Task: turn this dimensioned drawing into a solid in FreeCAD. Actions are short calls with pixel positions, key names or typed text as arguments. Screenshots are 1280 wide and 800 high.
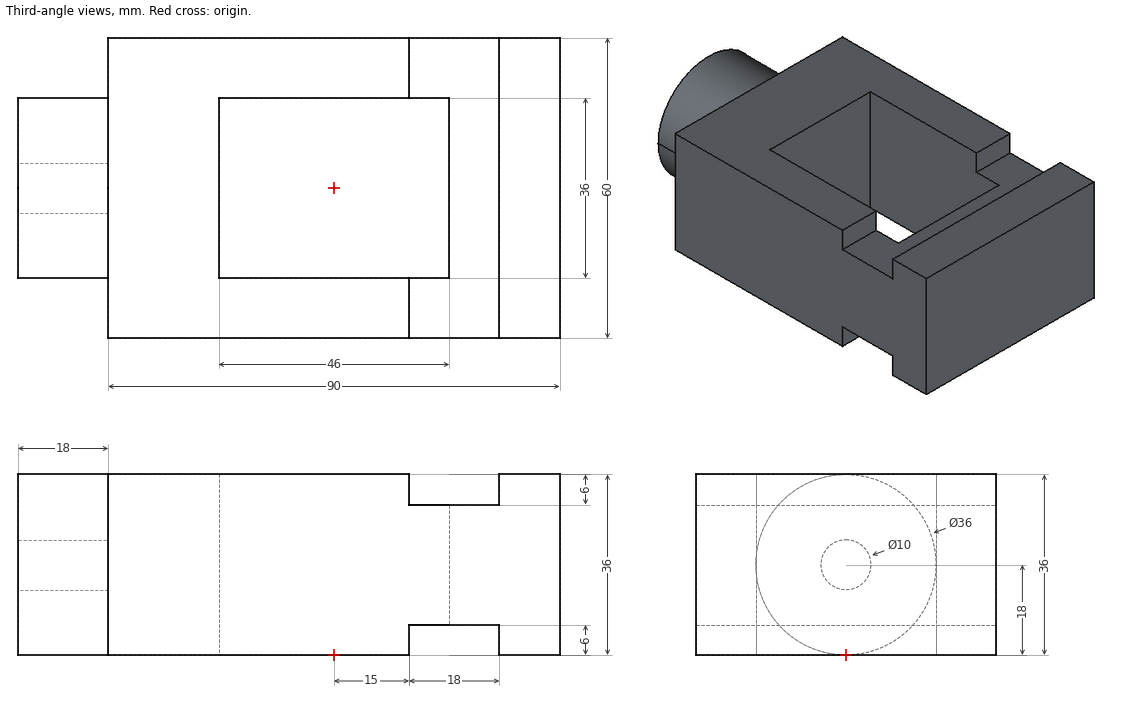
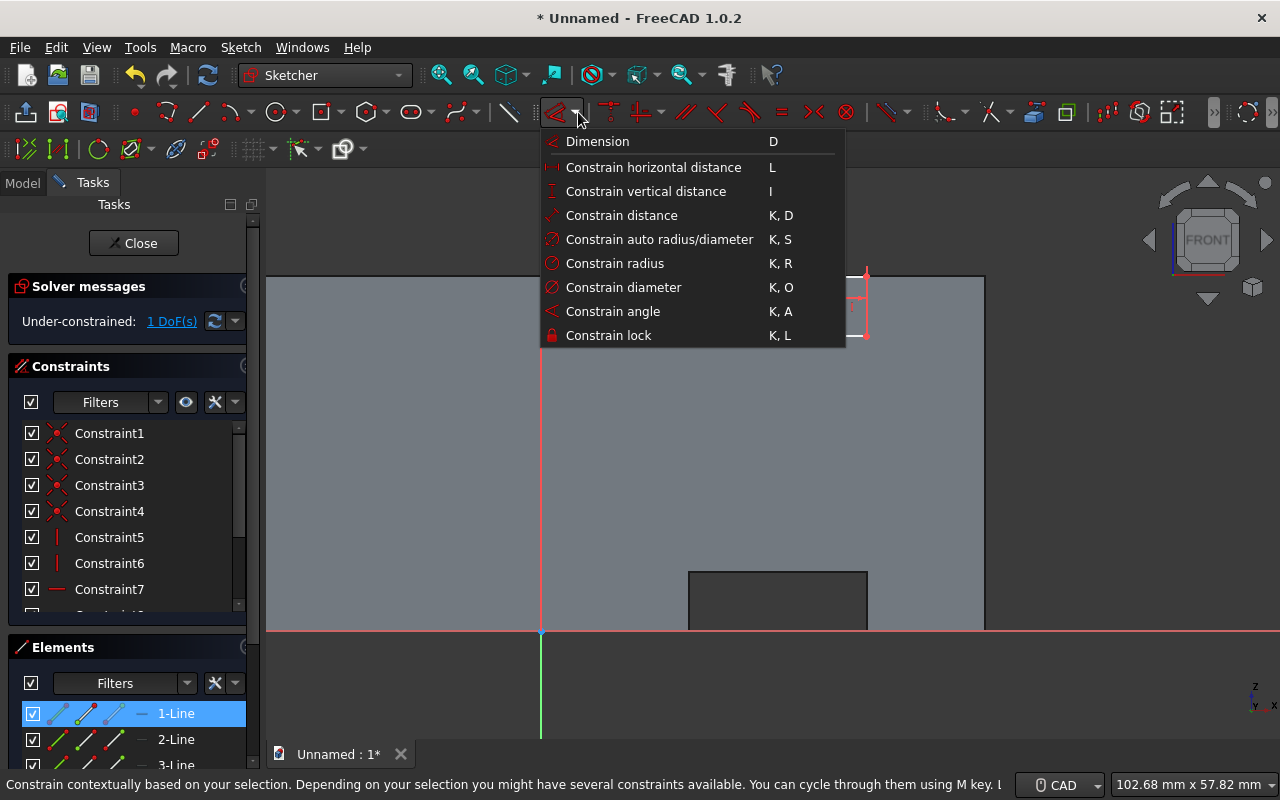
click(693, 191)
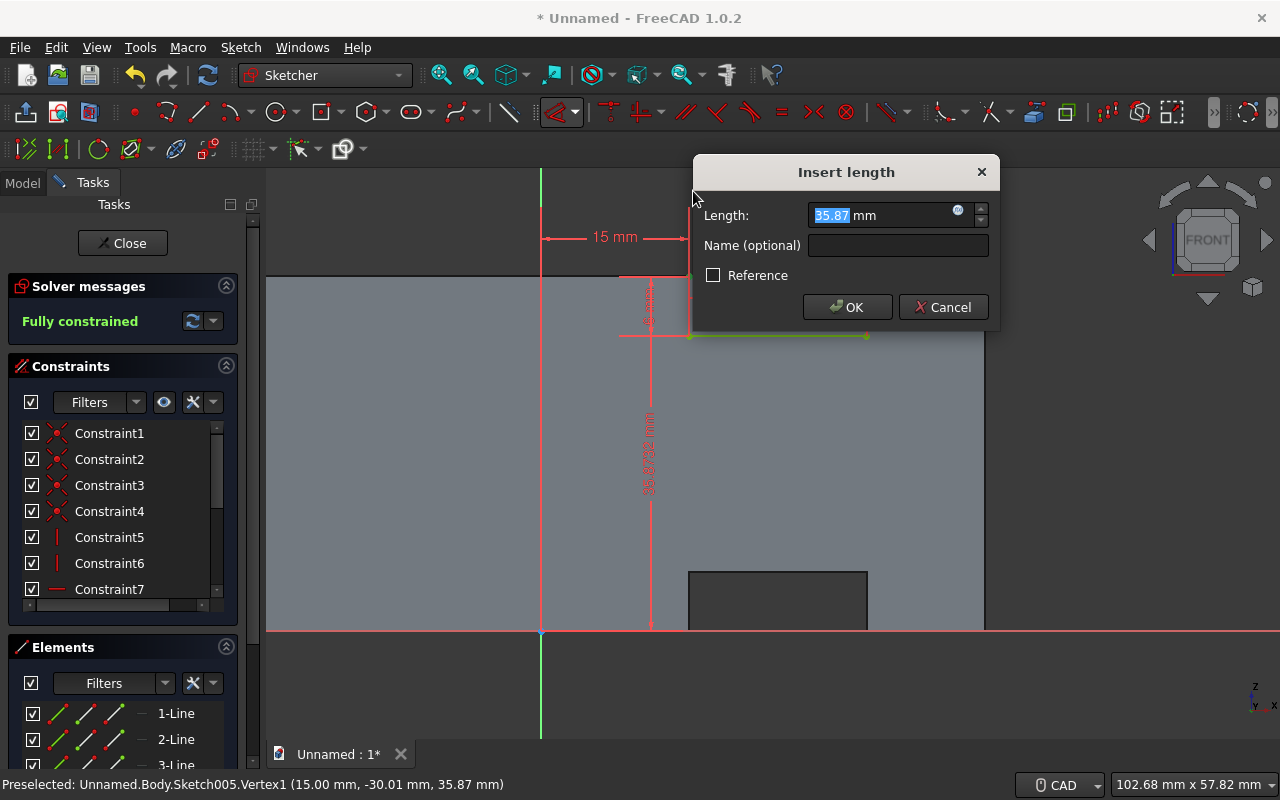
text(36)
key(Return)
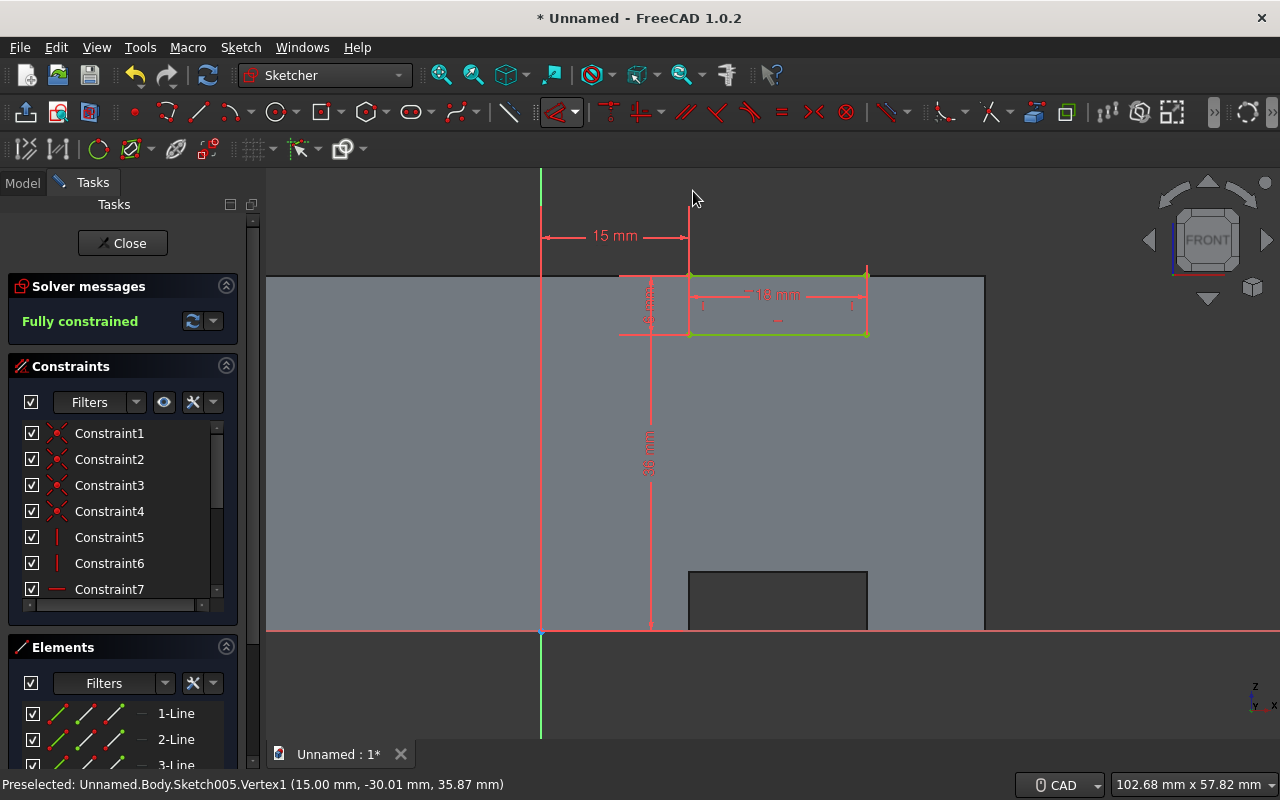
click(123, 243)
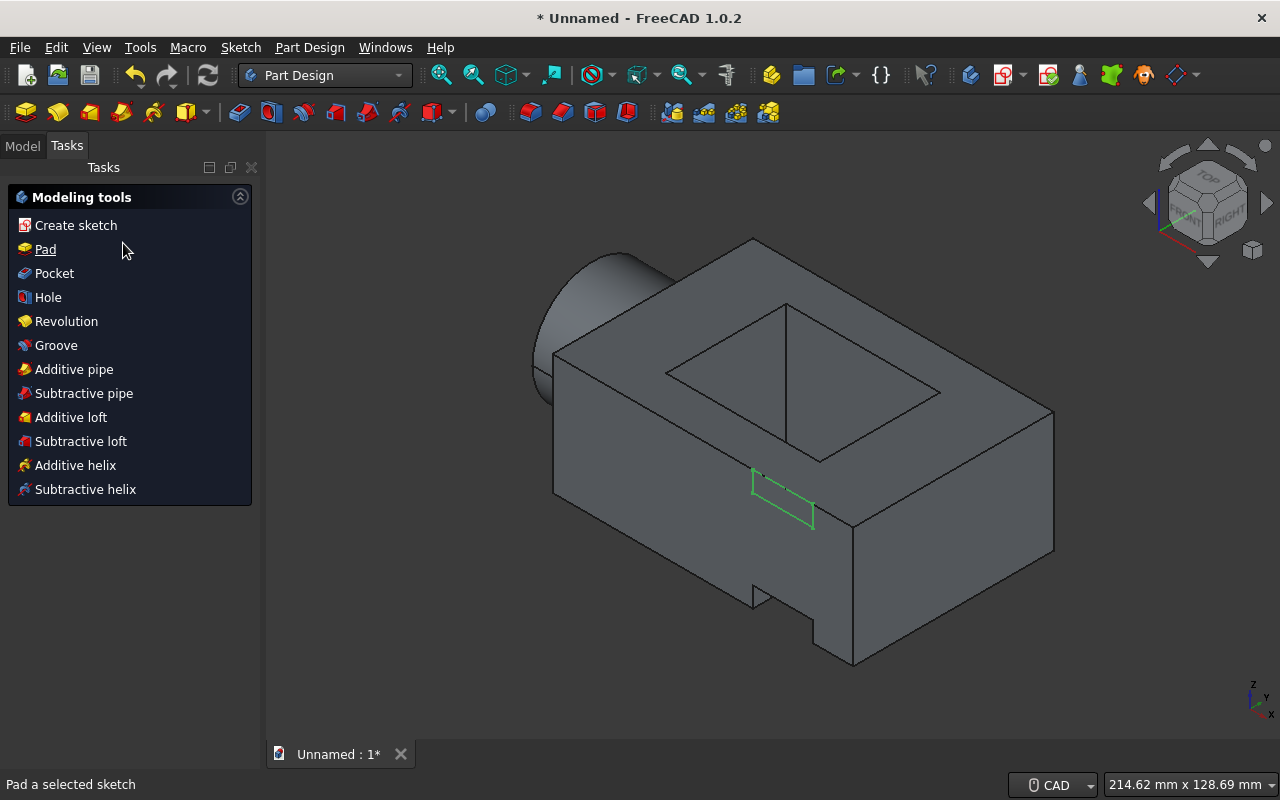
click(240, 112)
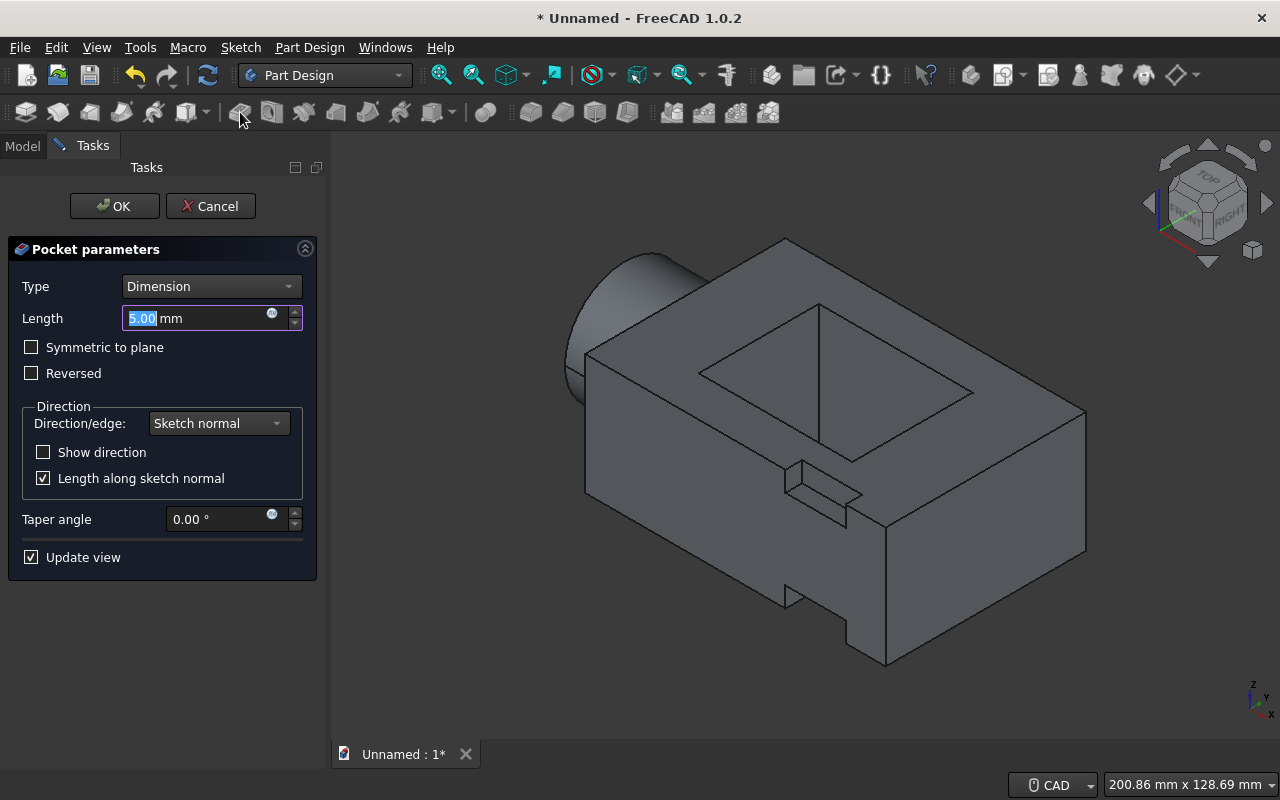
click(212, 286)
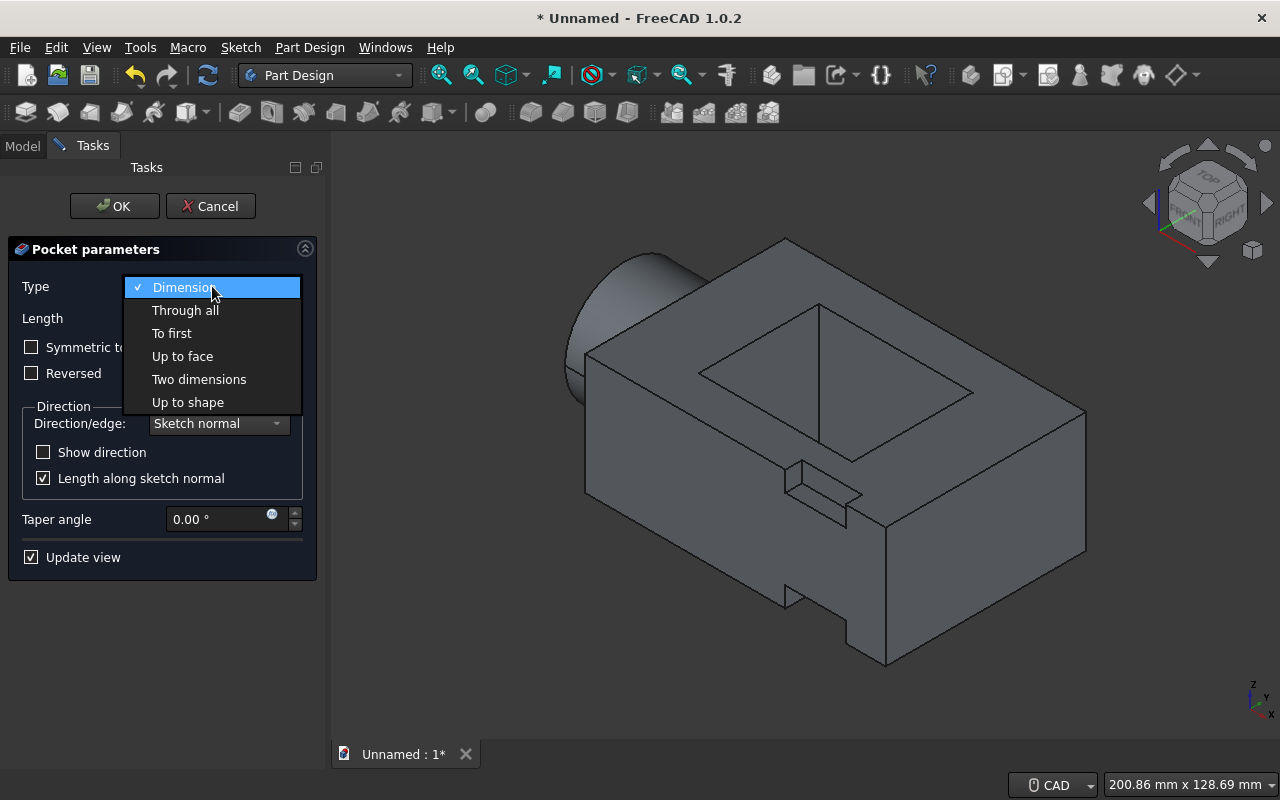
click(212, 310)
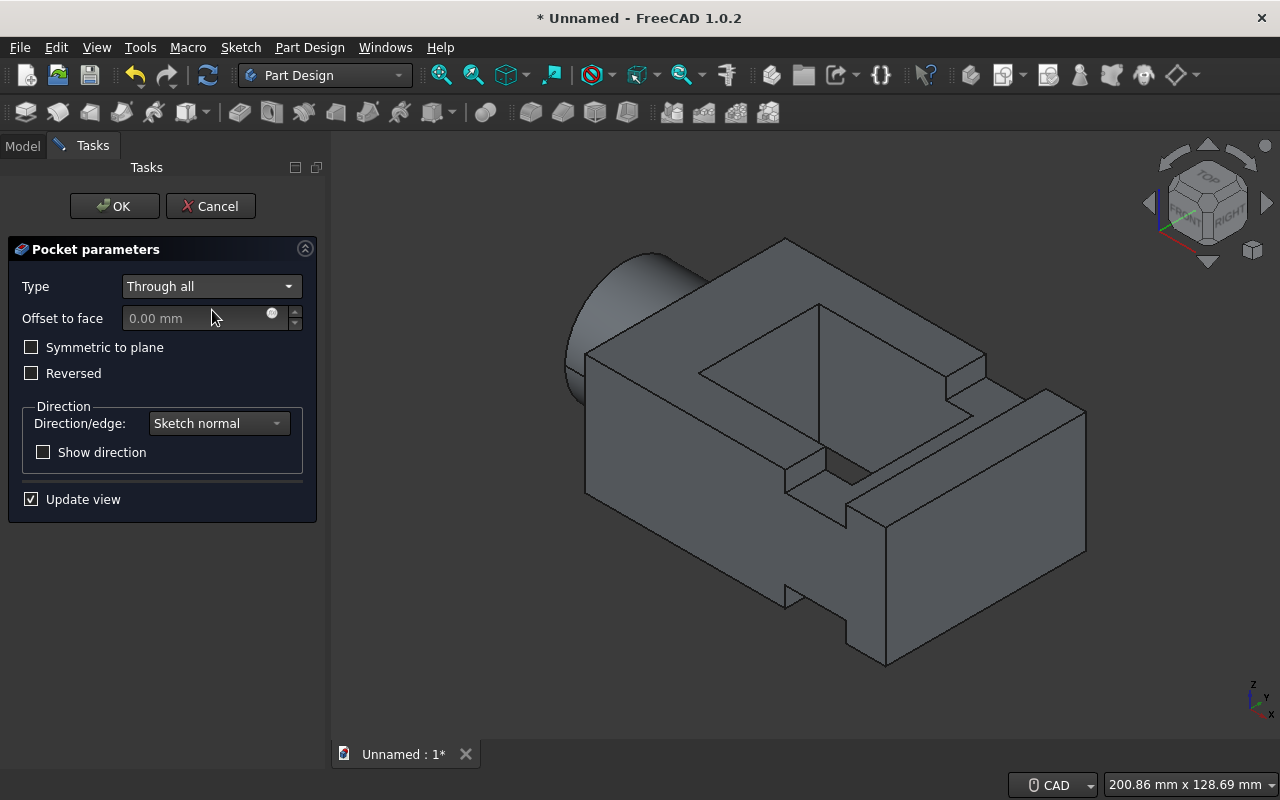
click(115, 206)